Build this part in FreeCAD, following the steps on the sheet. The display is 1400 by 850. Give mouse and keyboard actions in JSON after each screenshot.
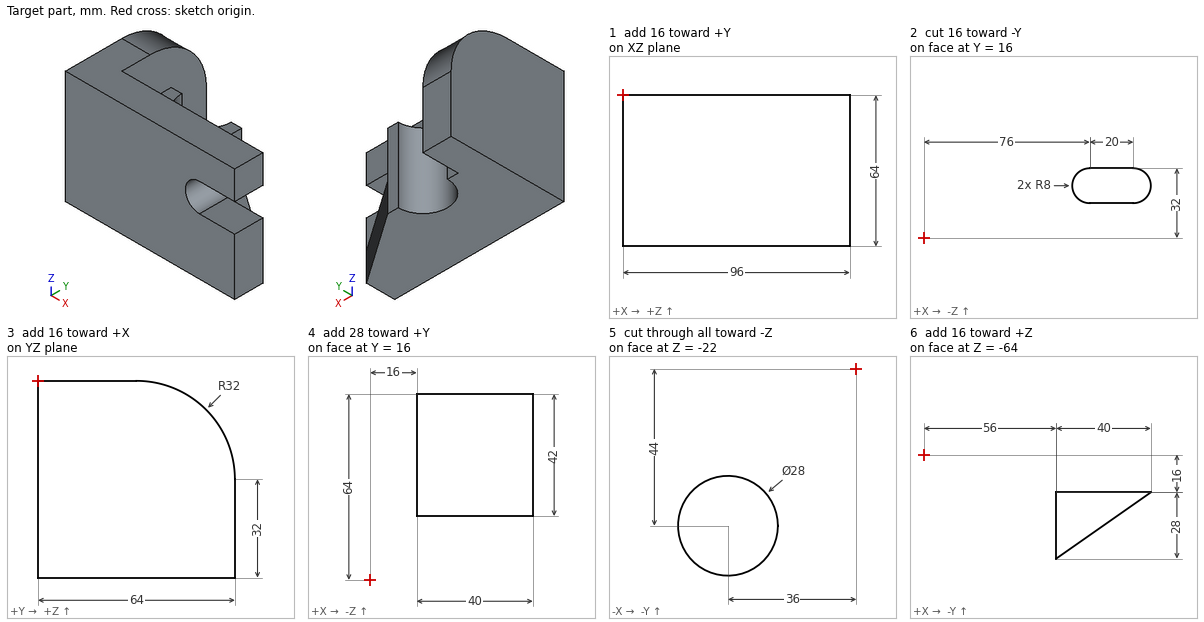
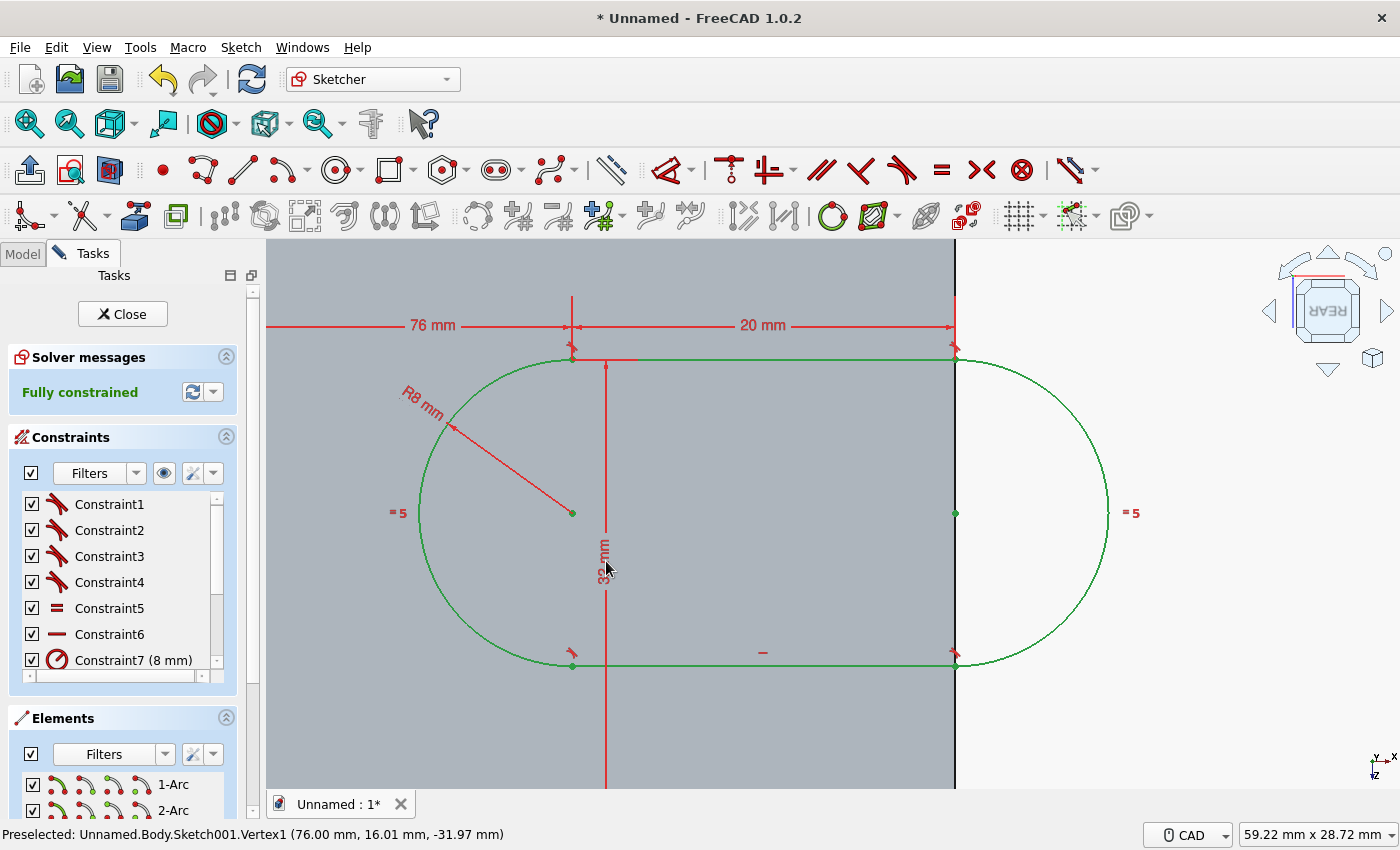
{"action": "left_click", "coordinate": [123, 314]}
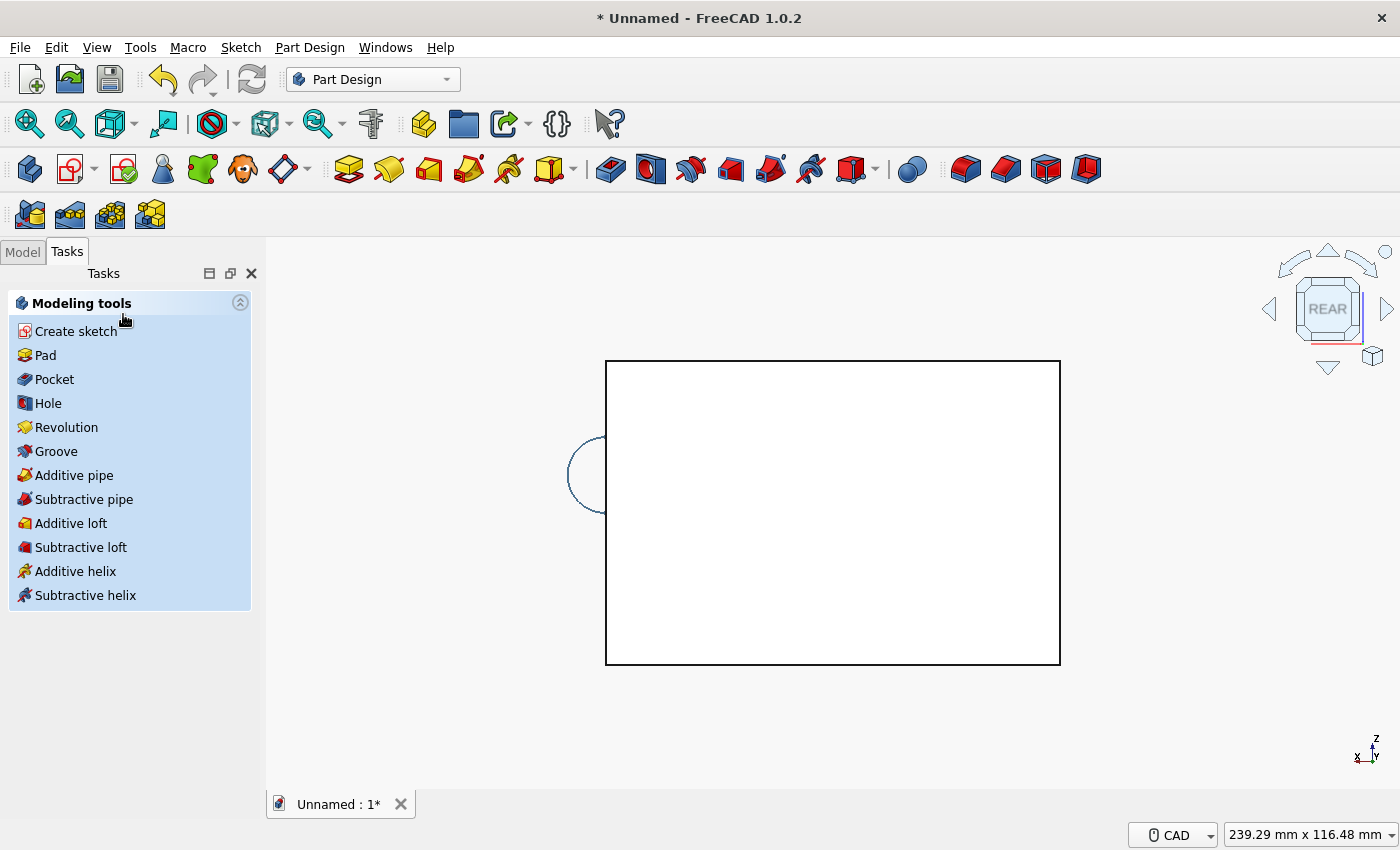
{"action": "left_click", "coordinate": [612, 170]}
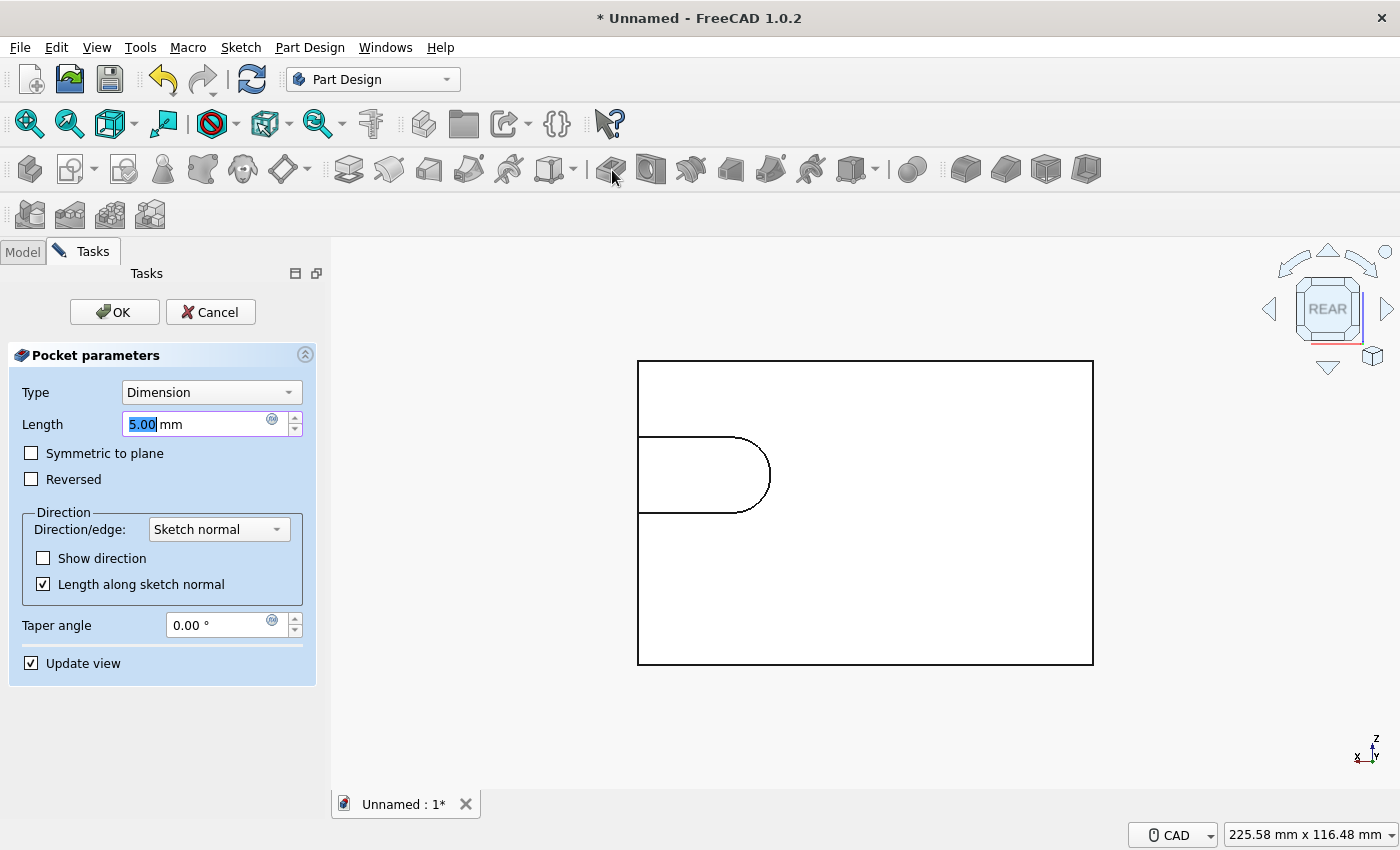
{"action": "type", "text": "16"}
{"action": "key", "text": "Tab"}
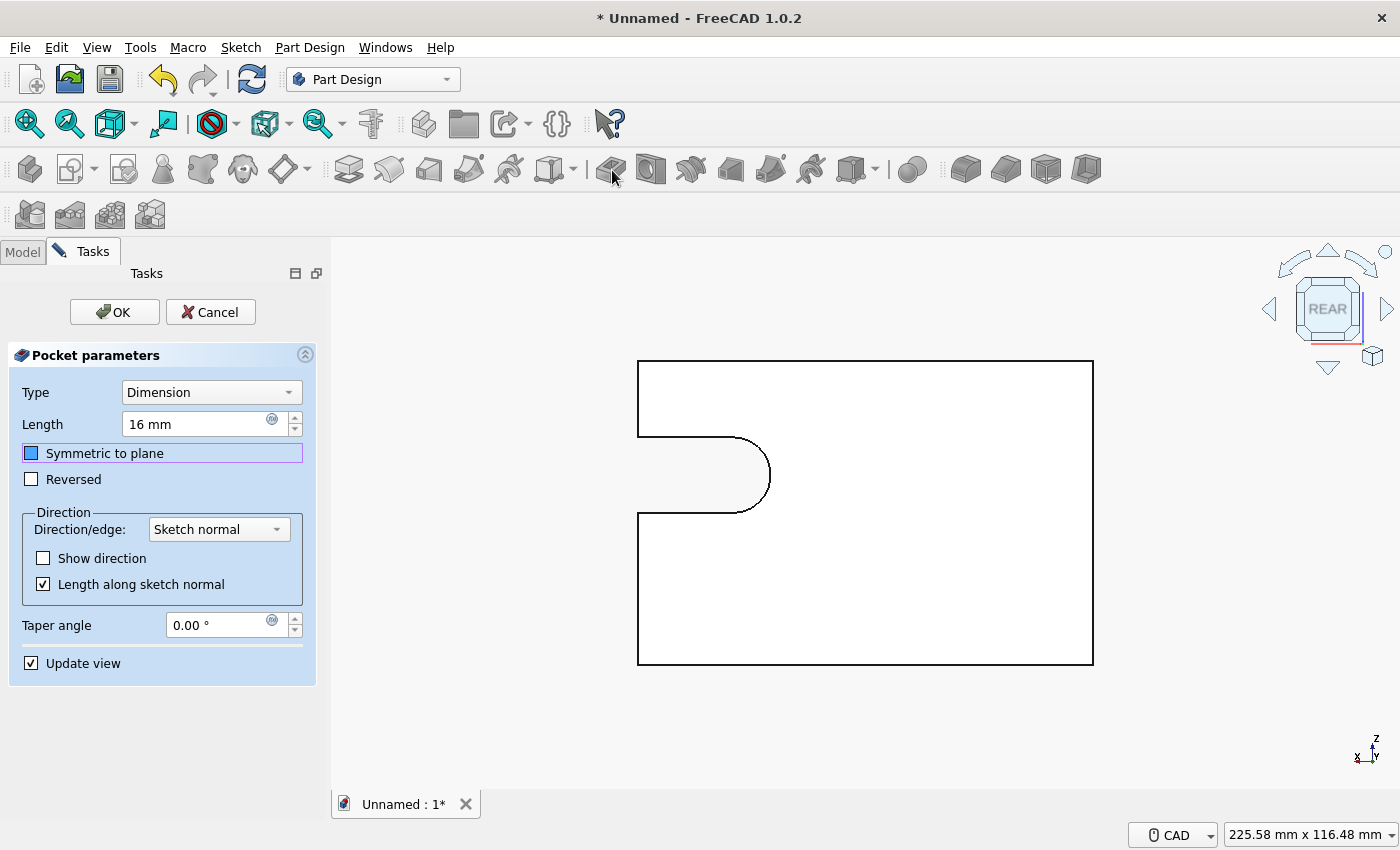
{"action": "left_click", "coordinate": [115, 312]}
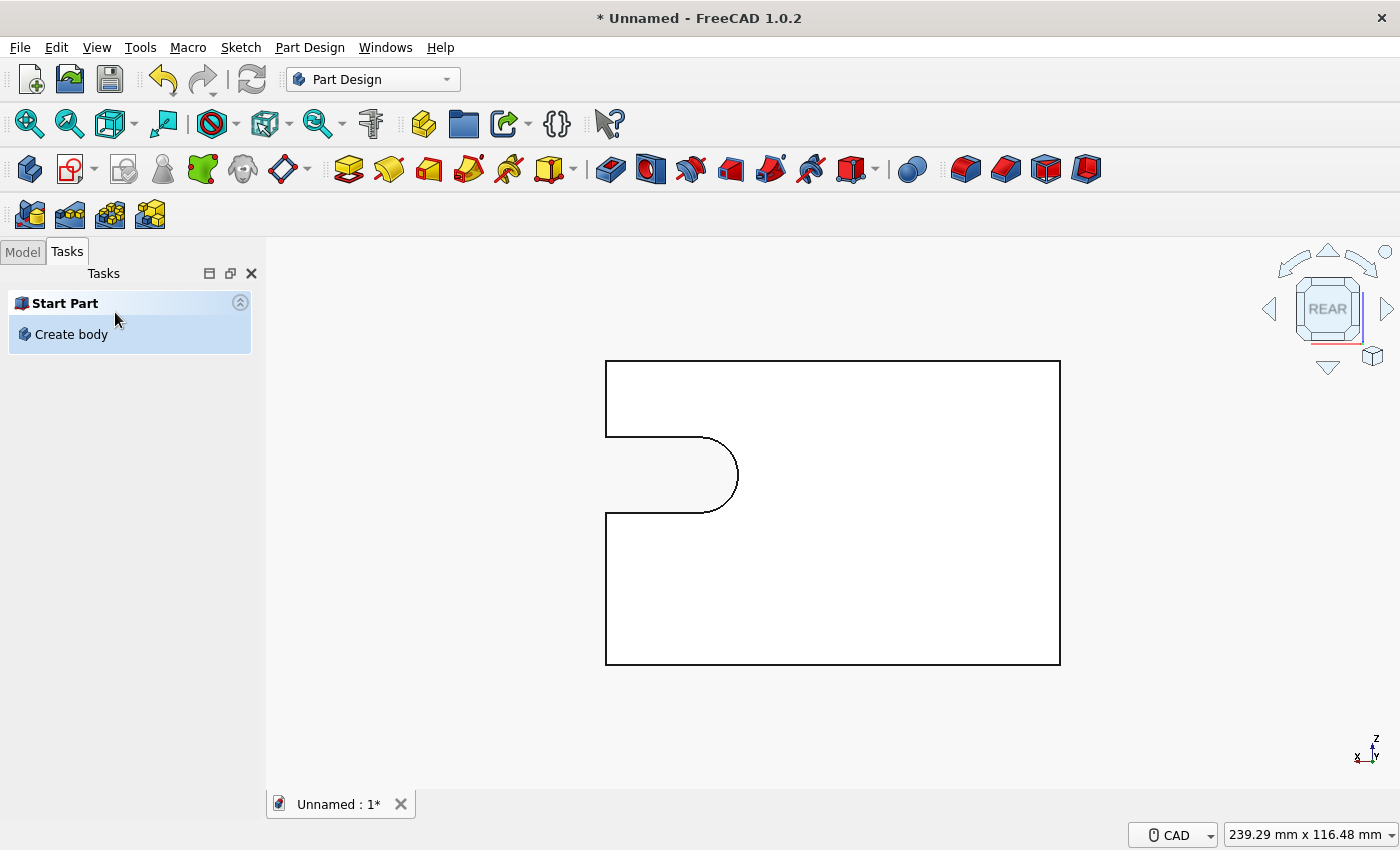
{"action": "left_click", "coordinate": [70, 170]}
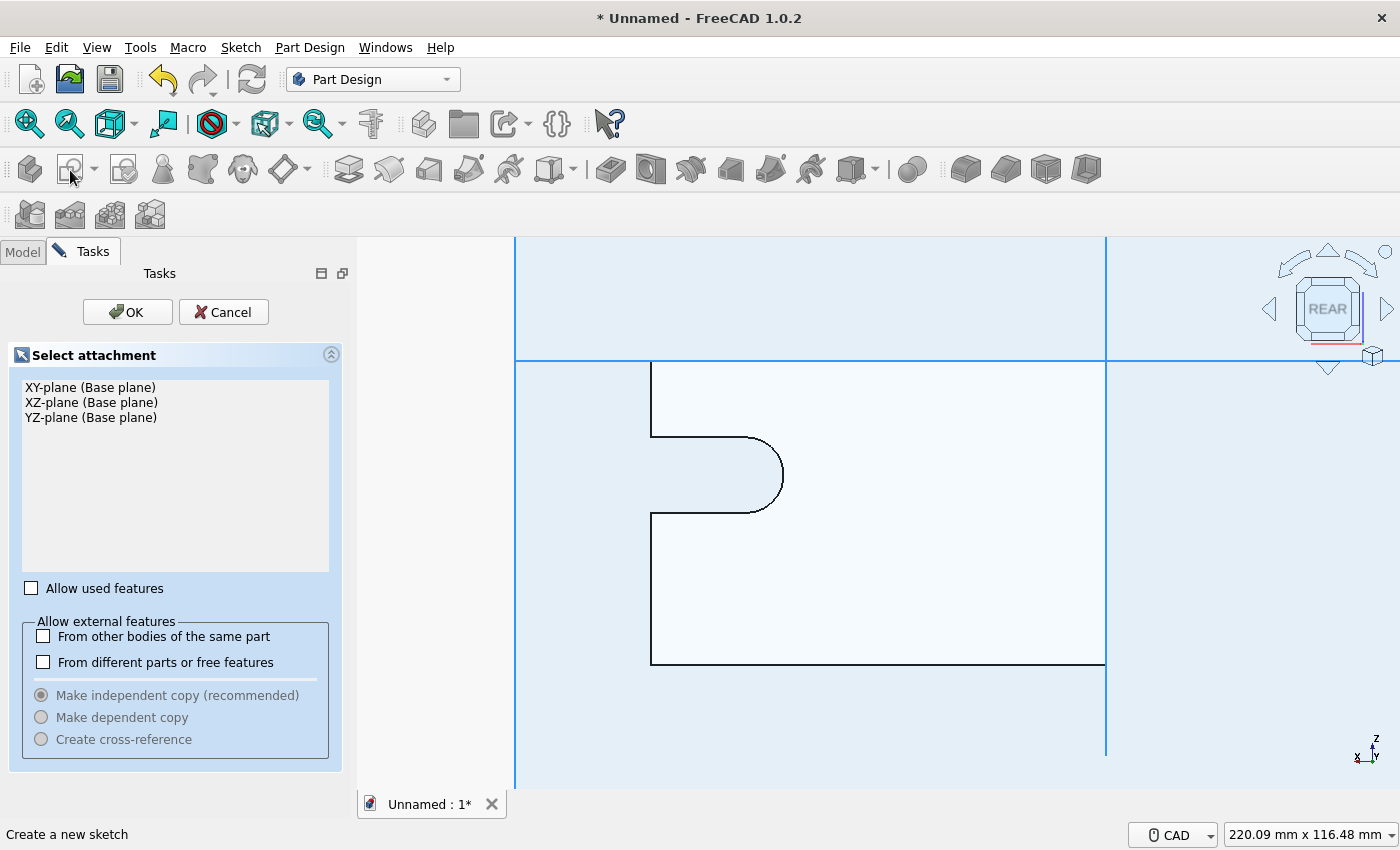
{"action": "left_click", "coordinate": [82, 418]}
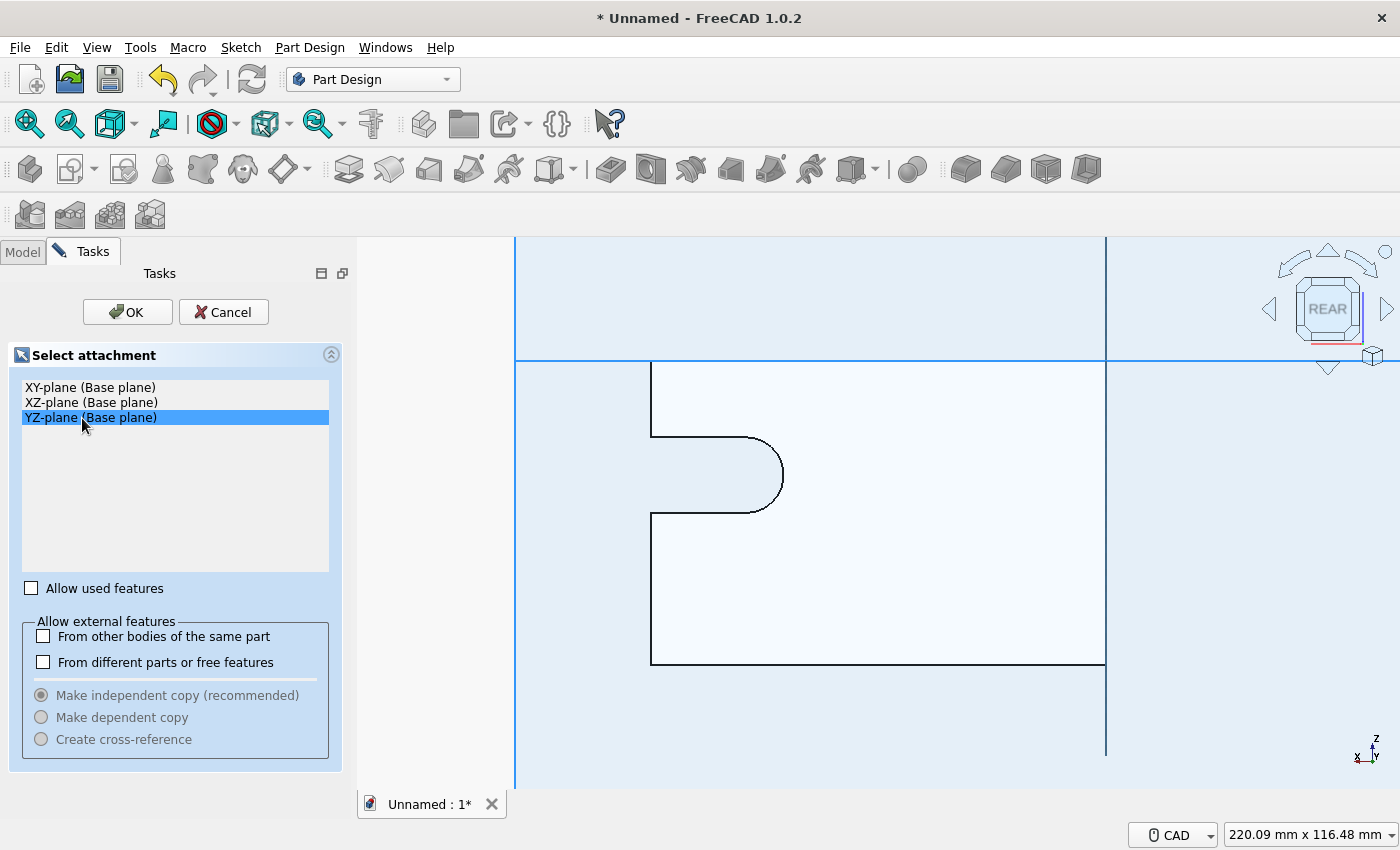
{"action": "left_click", "coordinate": [128, 312]}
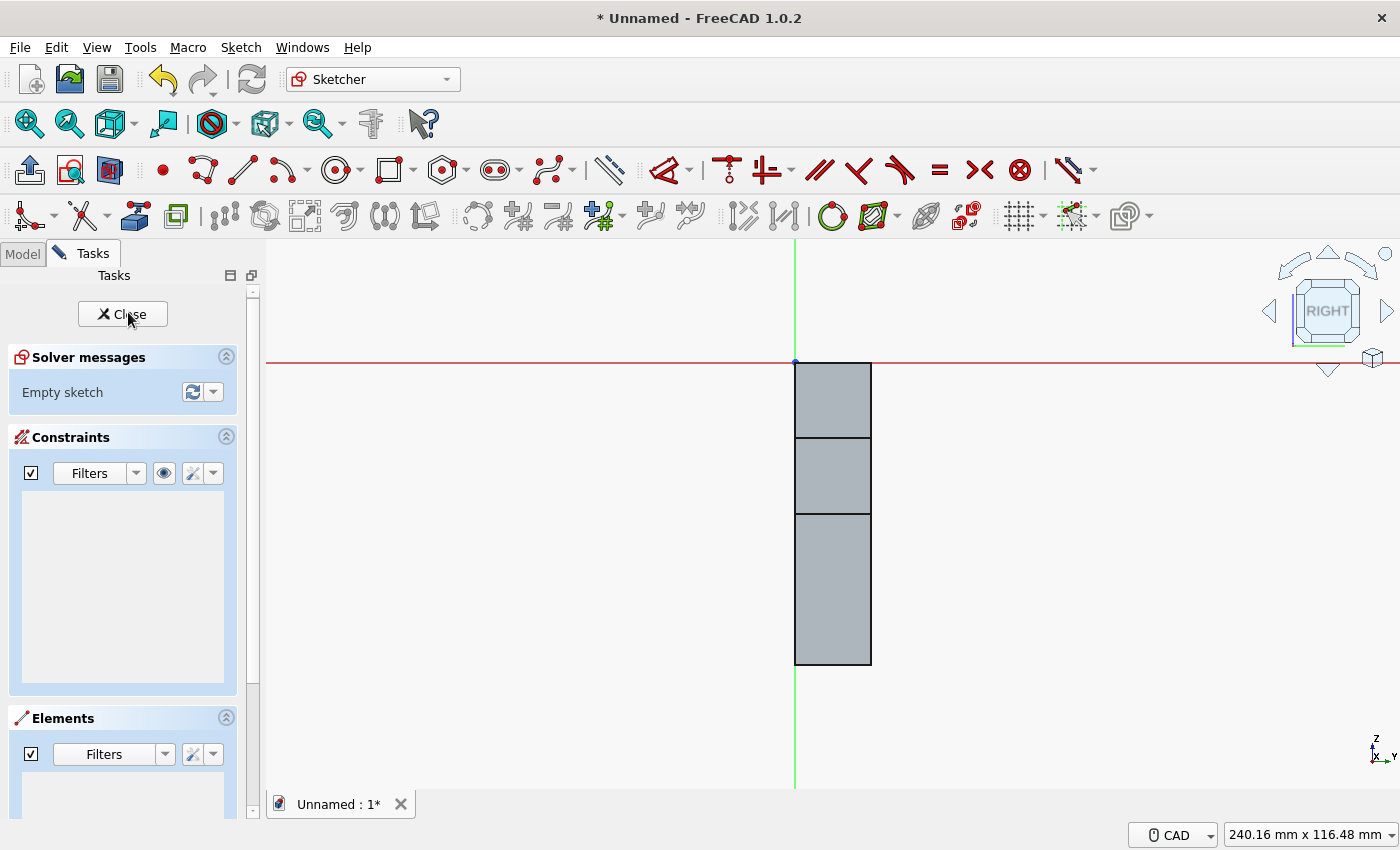
{"action": "left_click", "coordinate": [110, 170]}